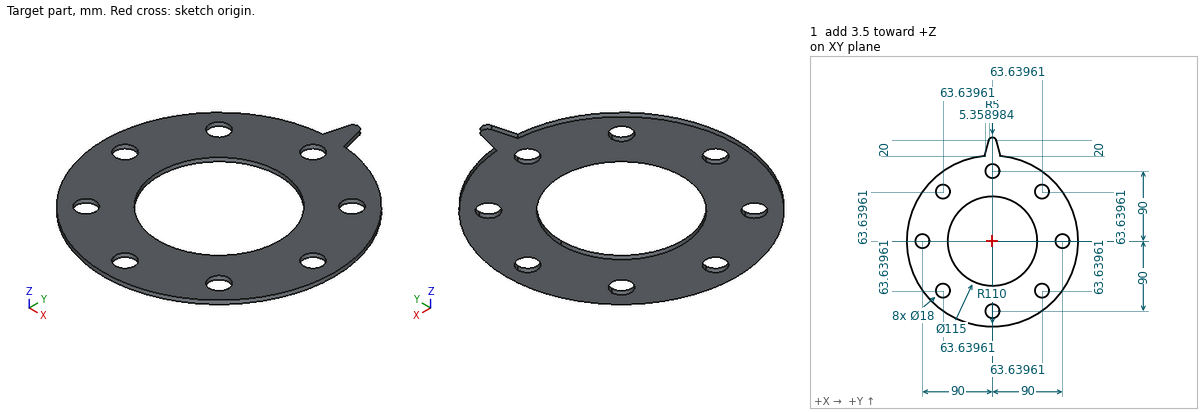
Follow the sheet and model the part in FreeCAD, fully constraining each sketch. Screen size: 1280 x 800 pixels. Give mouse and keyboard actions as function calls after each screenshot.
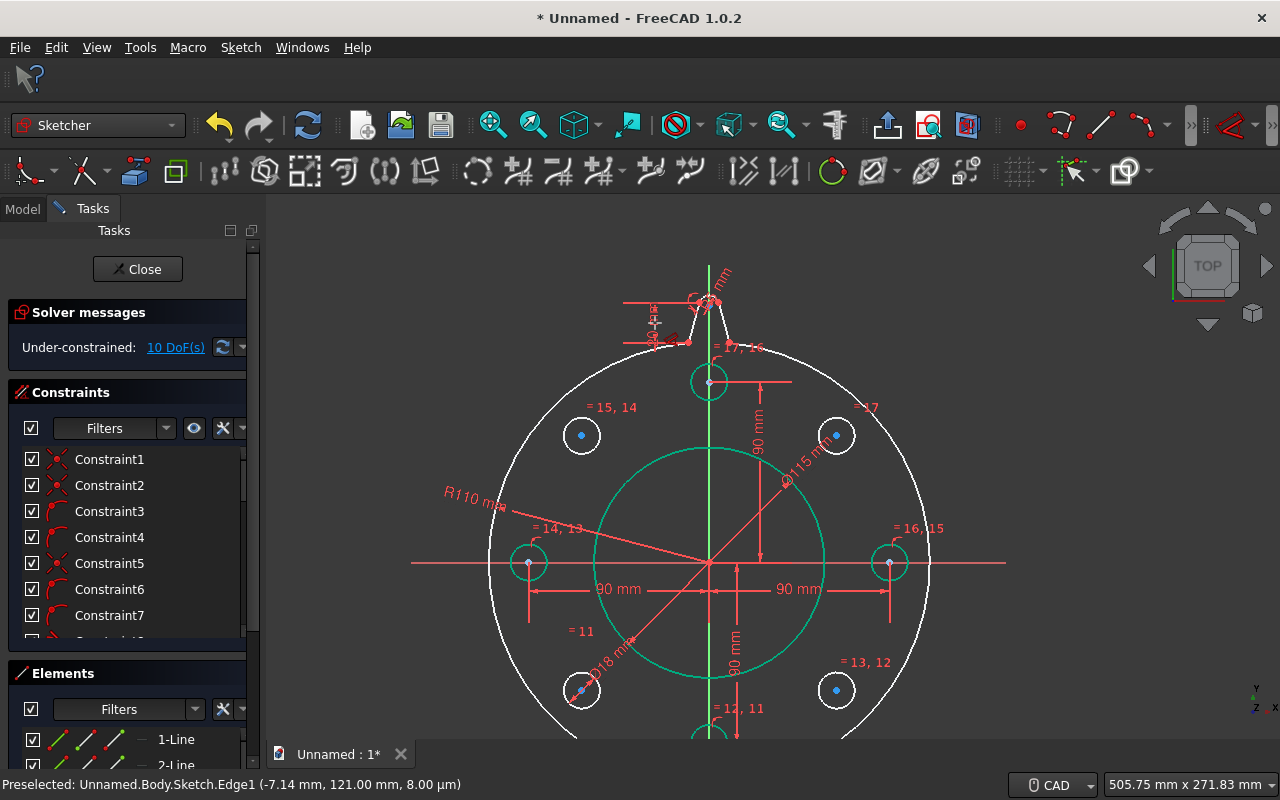
click(726, 331)
click(764, 323)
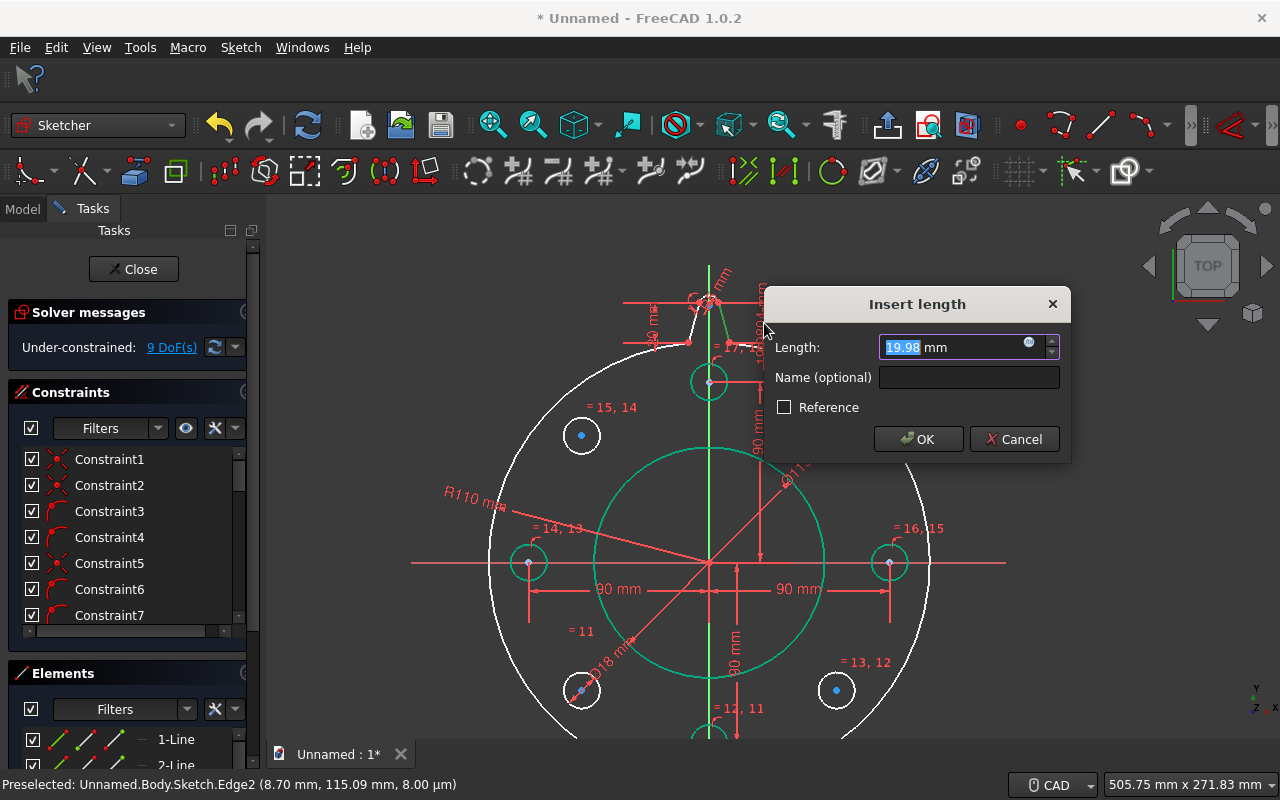
text(20)
key(Return)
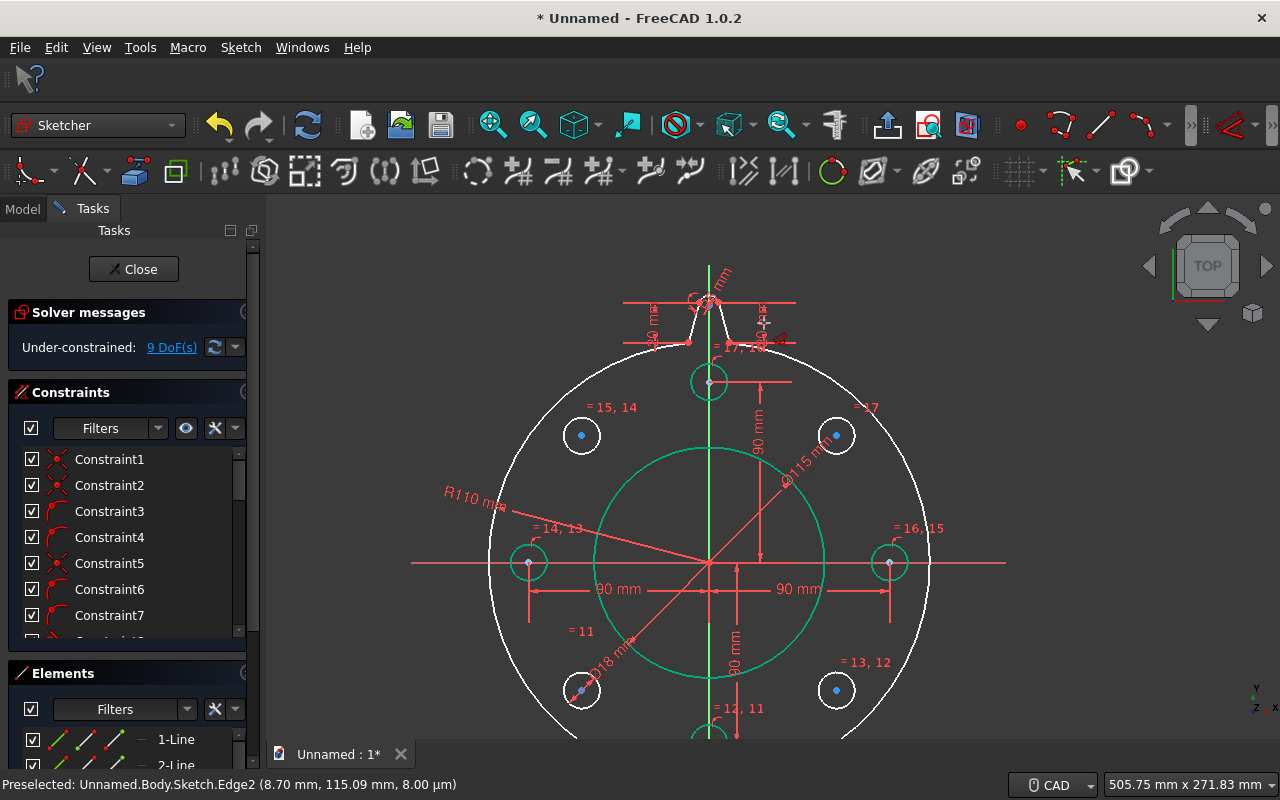
click(582, 691)
click(646, 529)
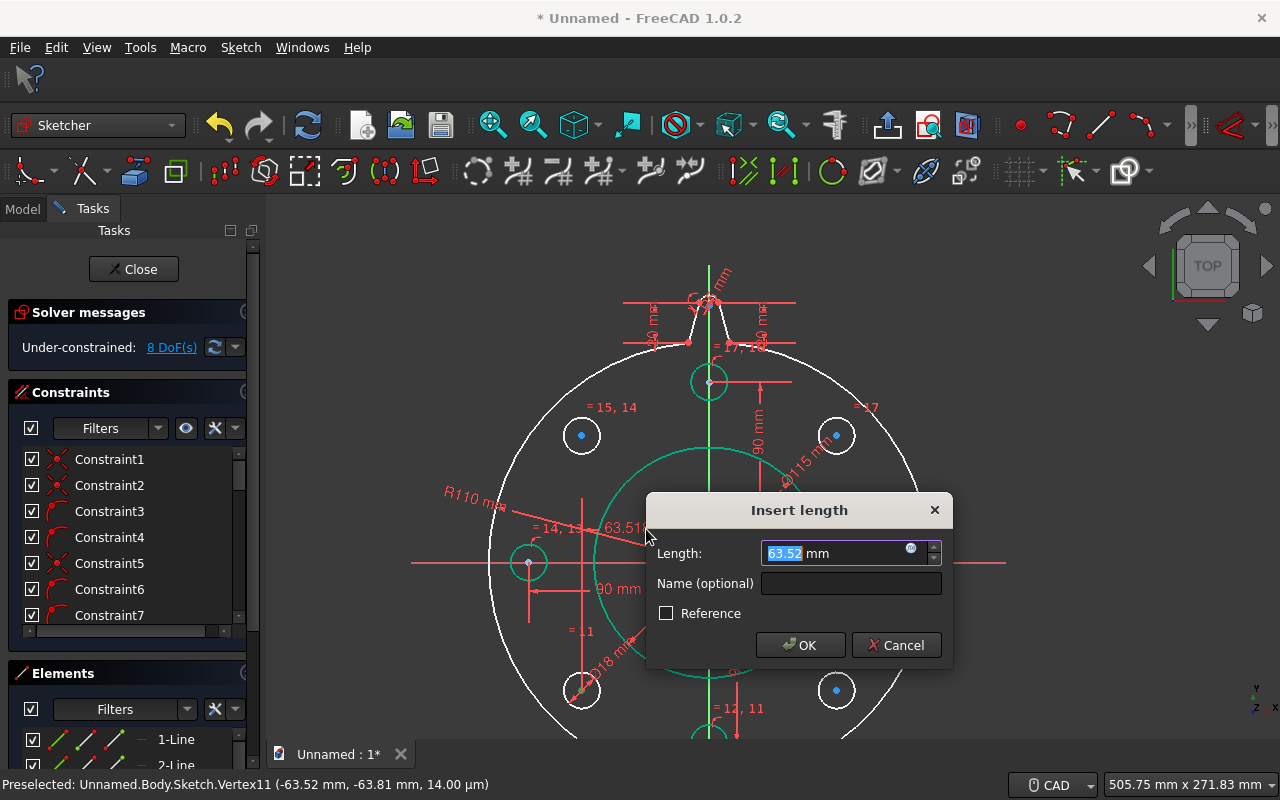
text(63.63961)
key(Return)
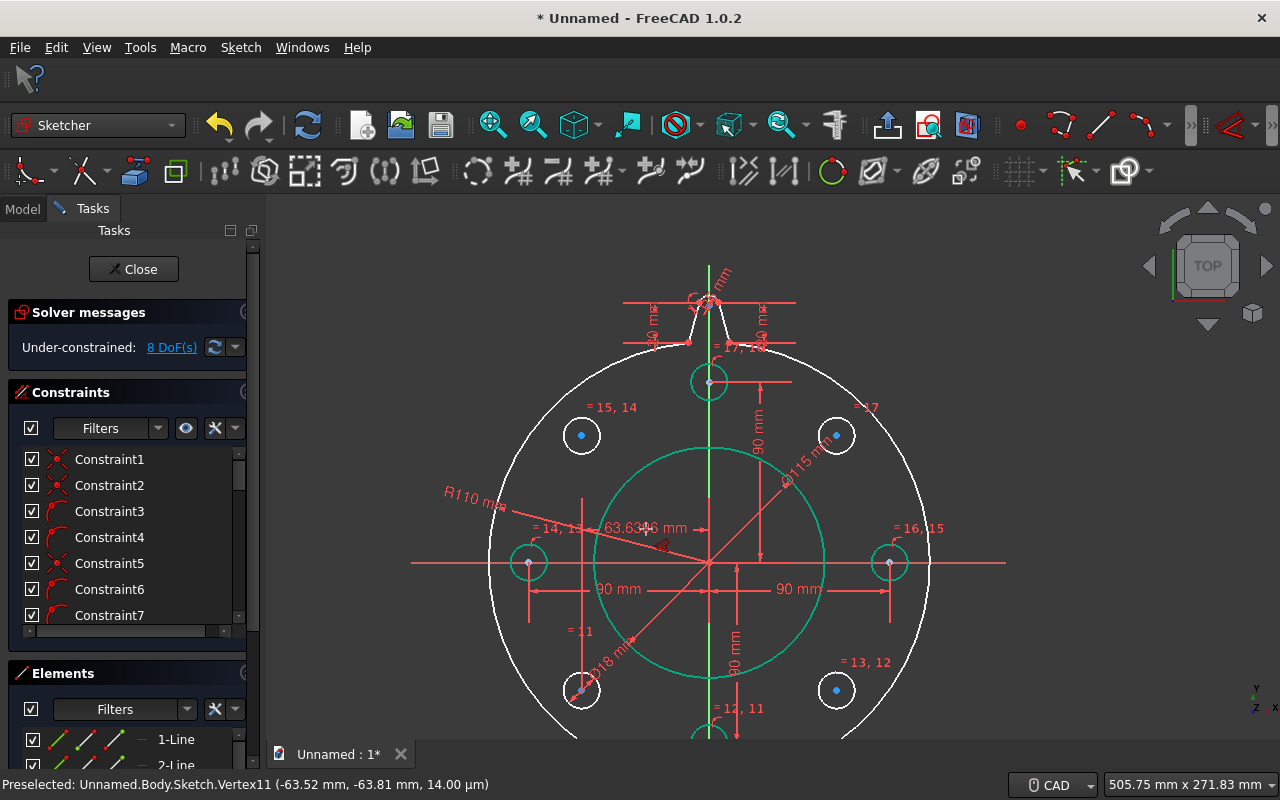
click(582, 691)
click(548, 627)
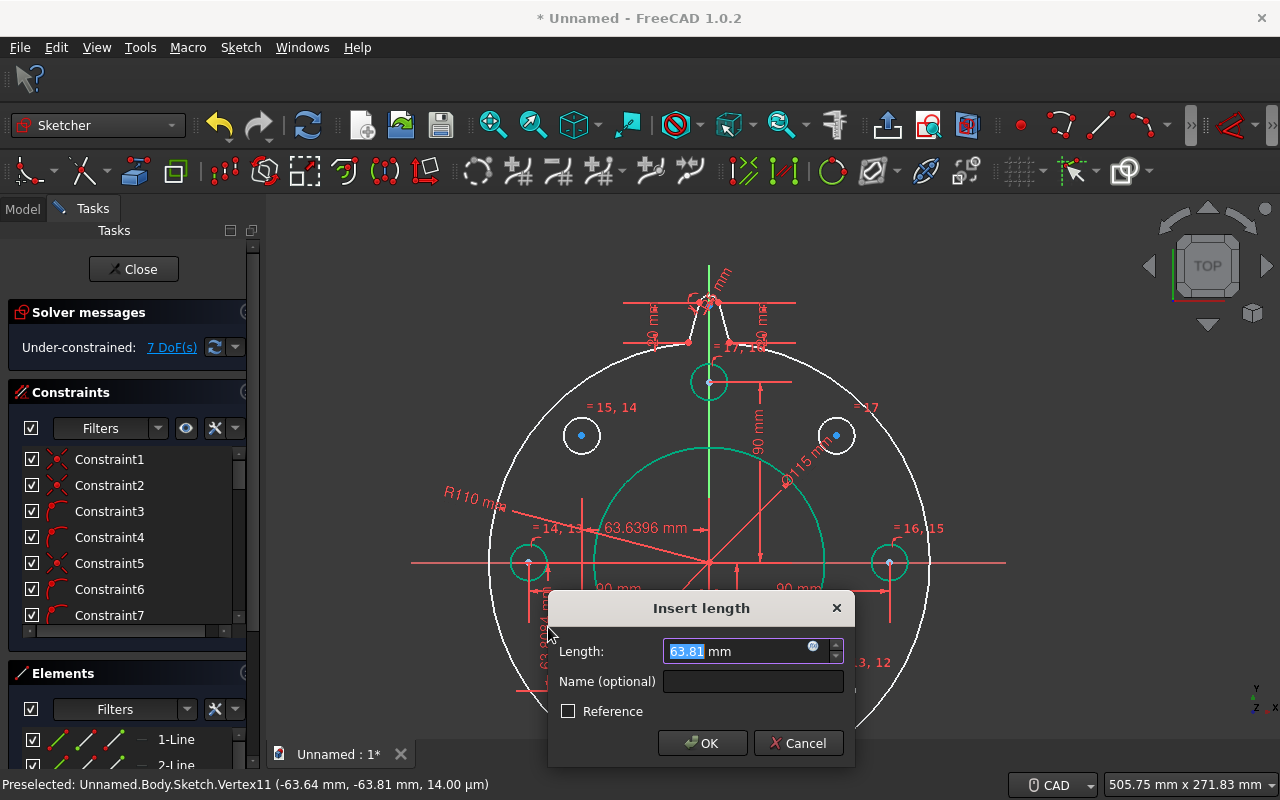
text(63.63961)
key(Return)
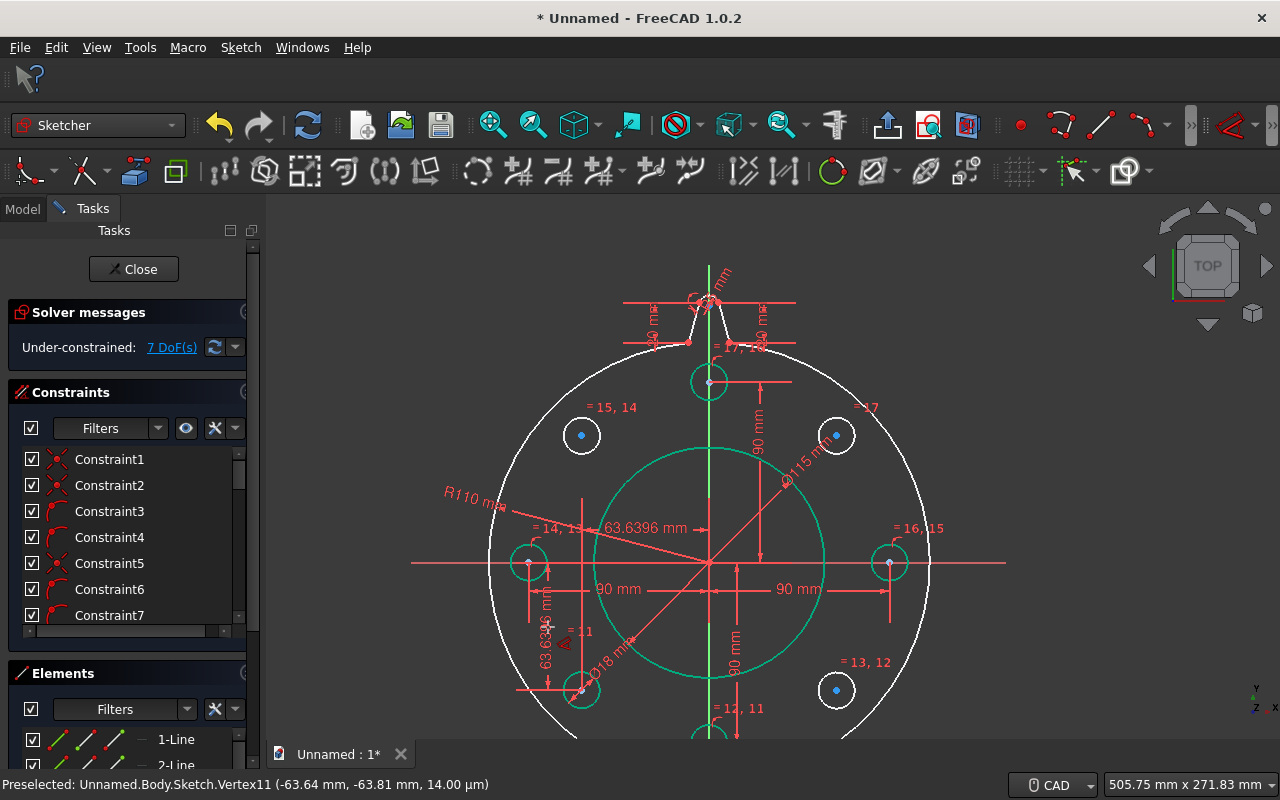
click(837, 691)
click(773, 529)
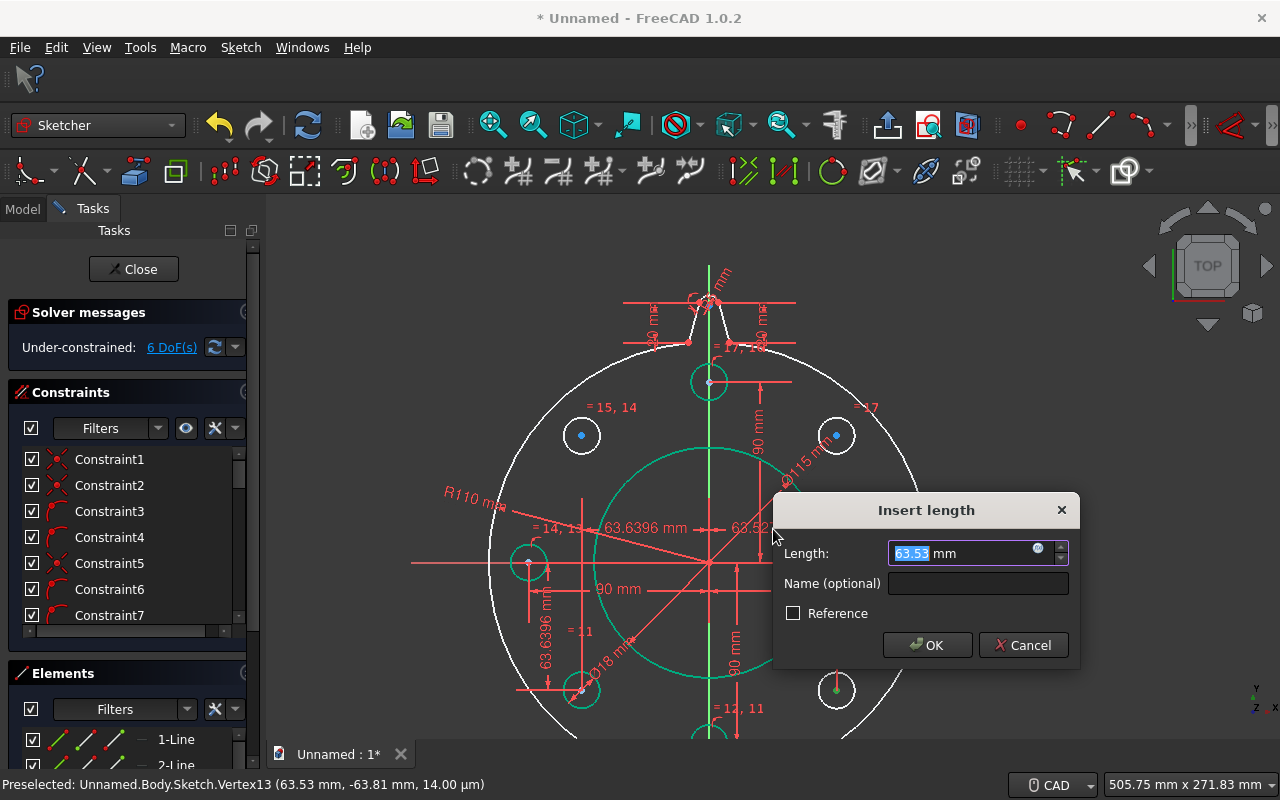
text(63.63961)
key(Return)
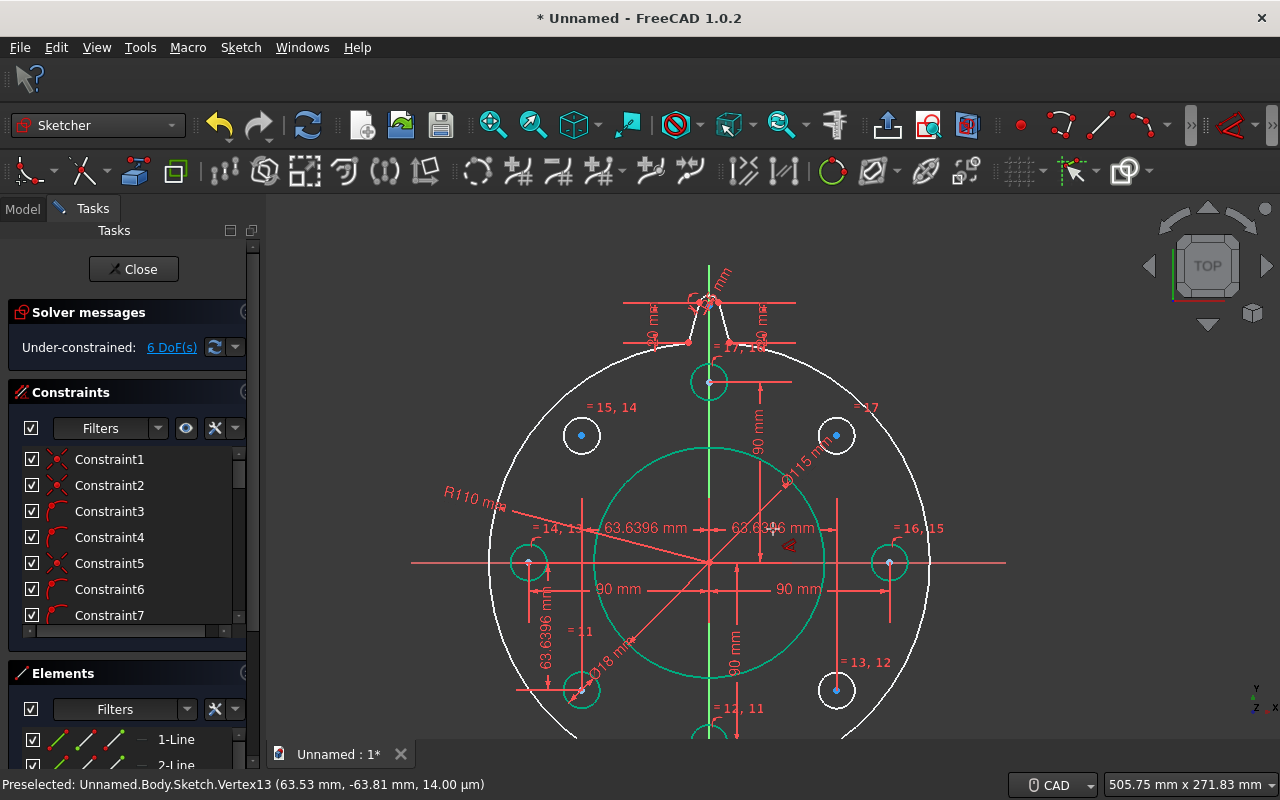
click(837, 691)
click(871, 627)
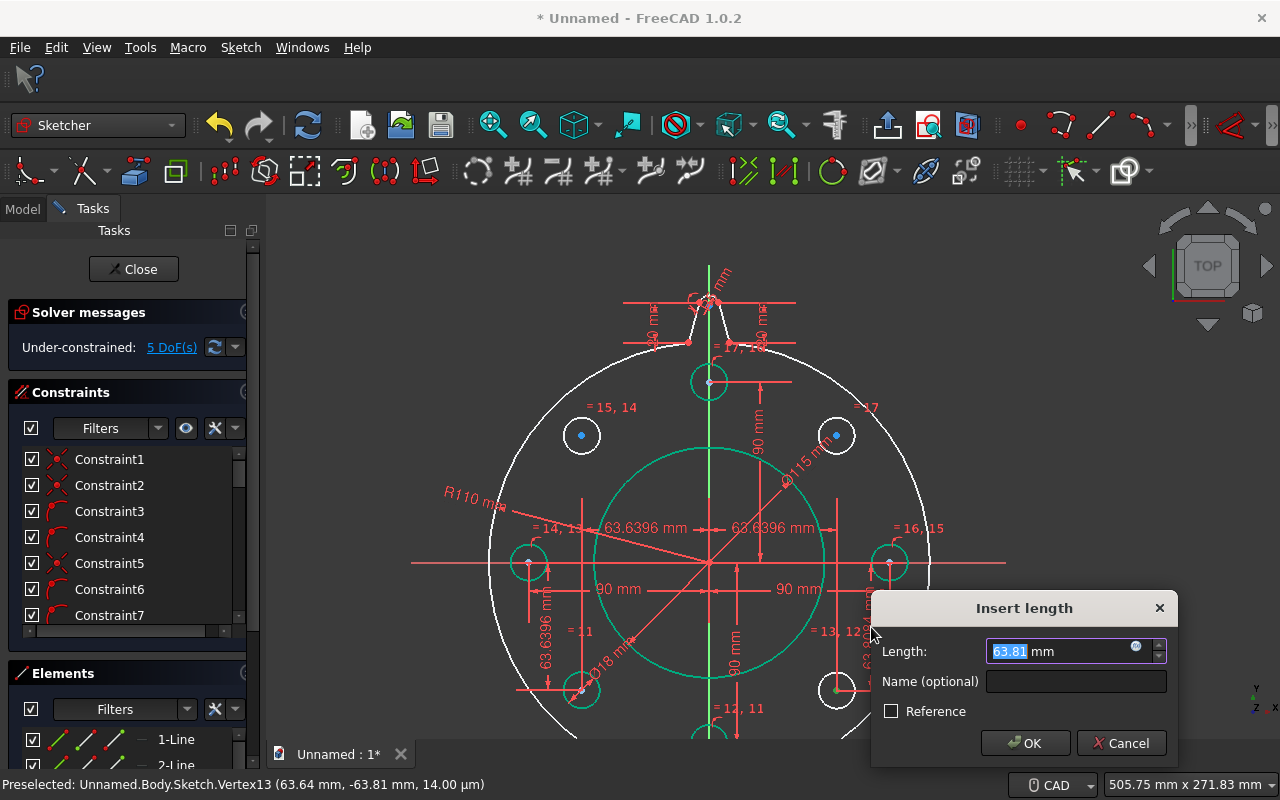
text(63.63961)
key(Return)